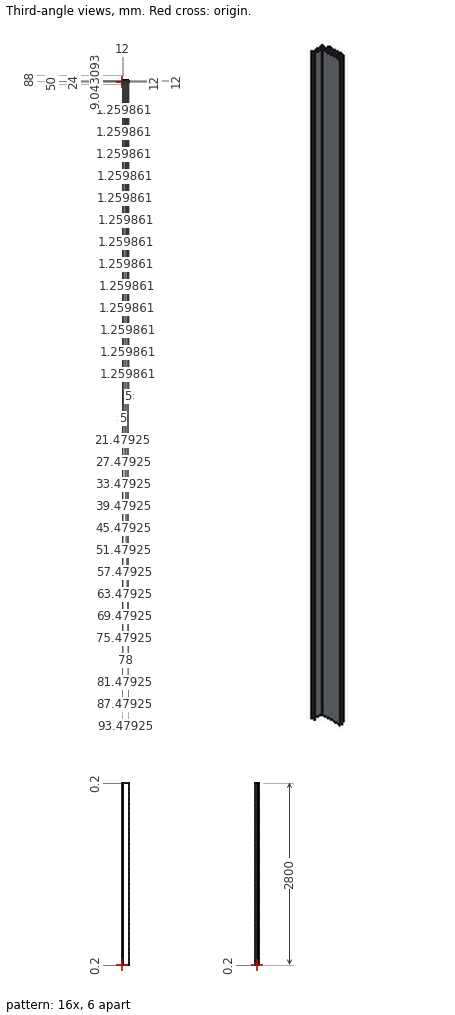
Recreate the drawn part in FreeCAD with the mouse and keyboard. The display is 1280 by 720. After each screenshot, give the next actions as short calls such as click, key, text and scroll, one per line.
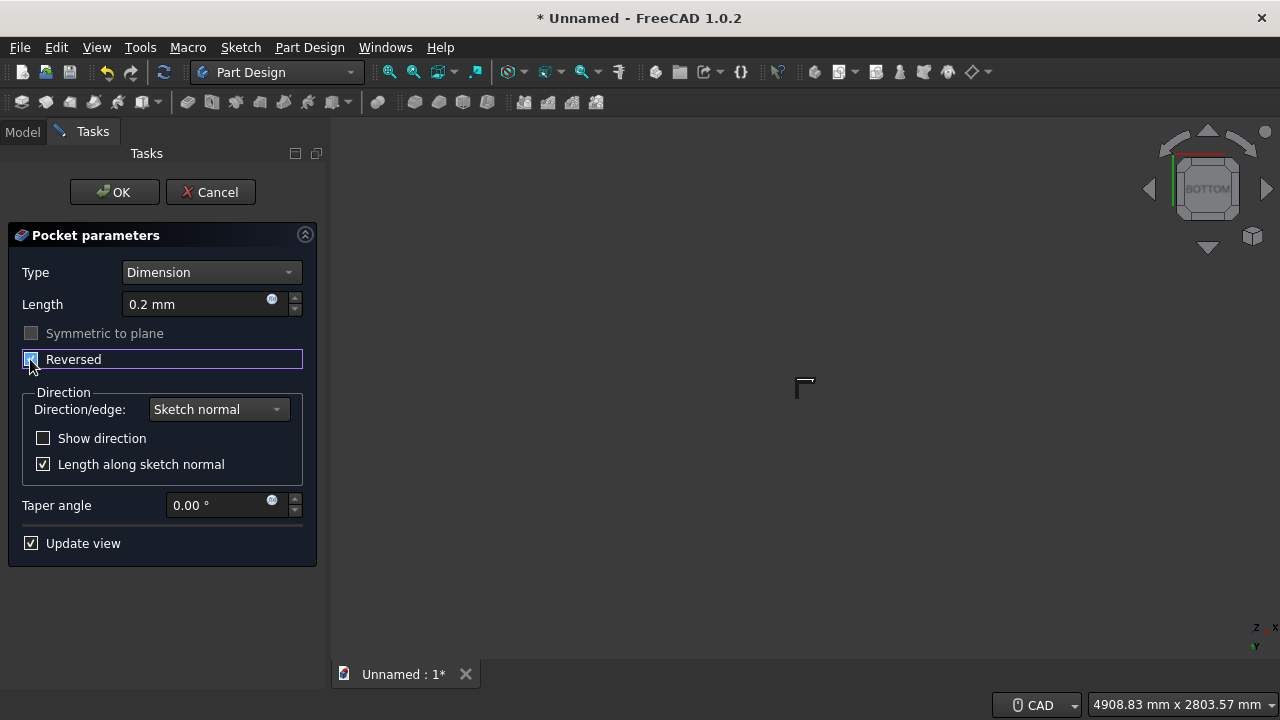
click(115, 192)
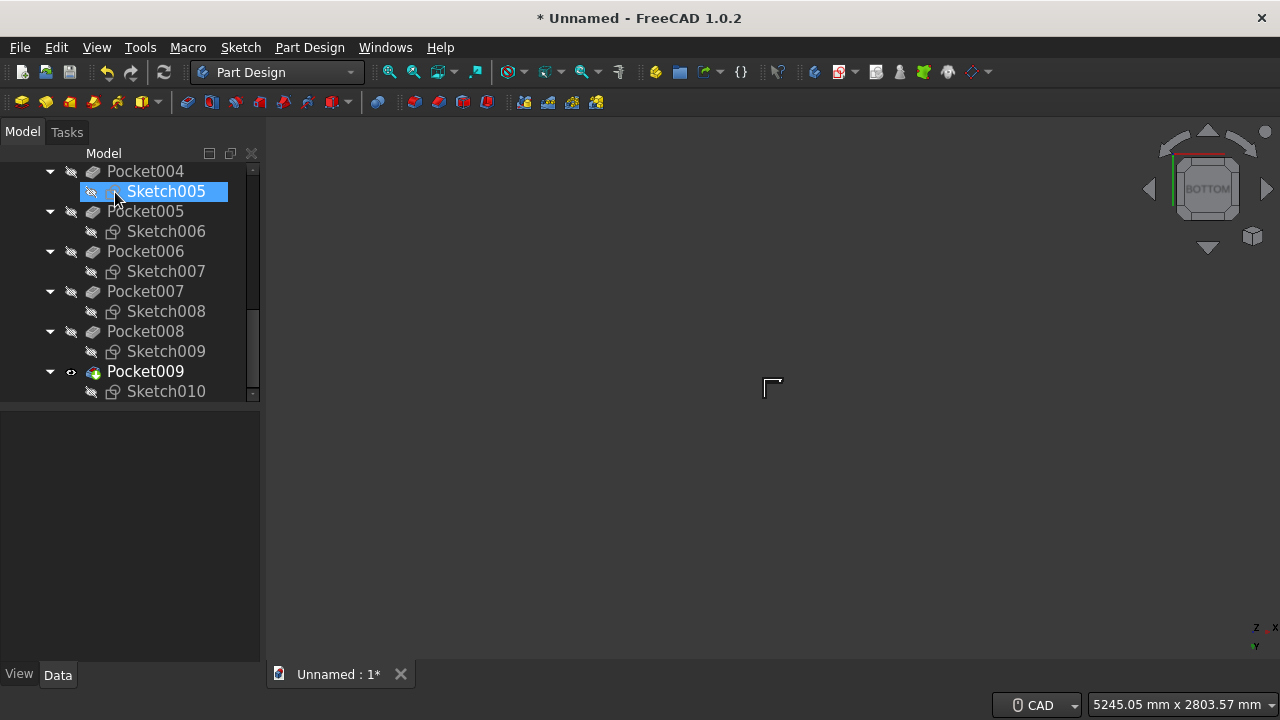
click(390, 72)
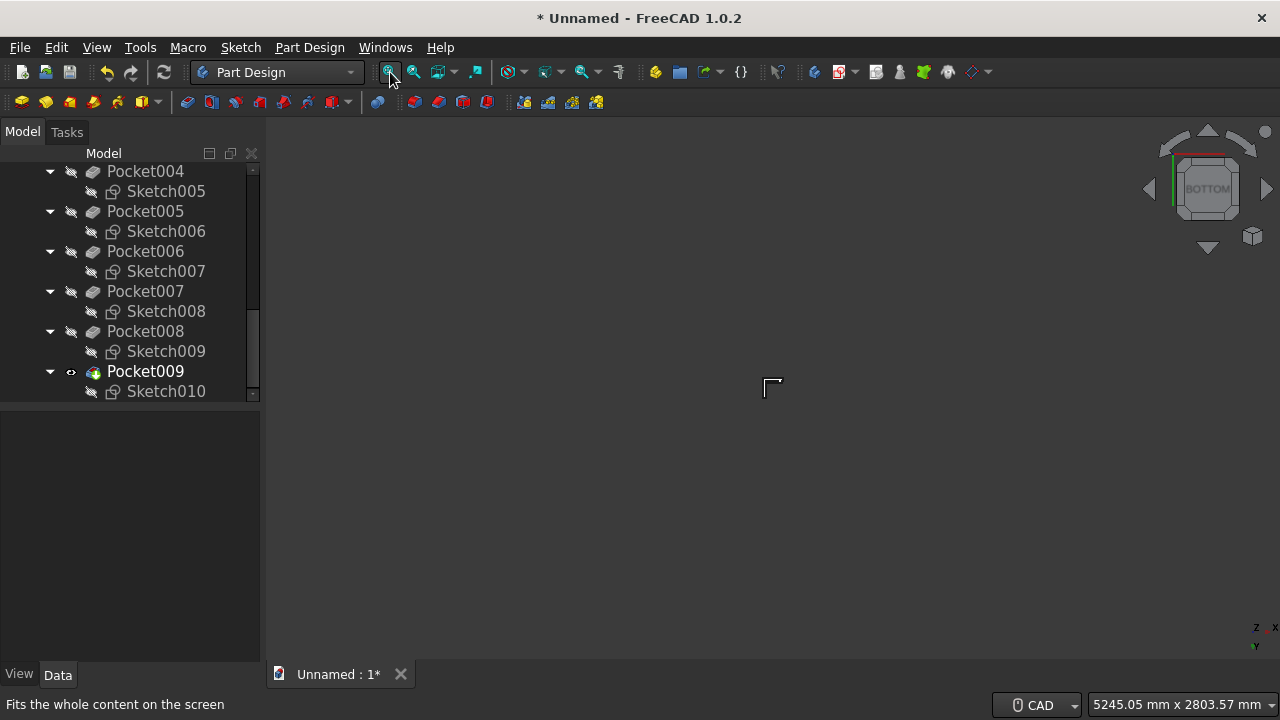
scroll(779, 379, up, 11)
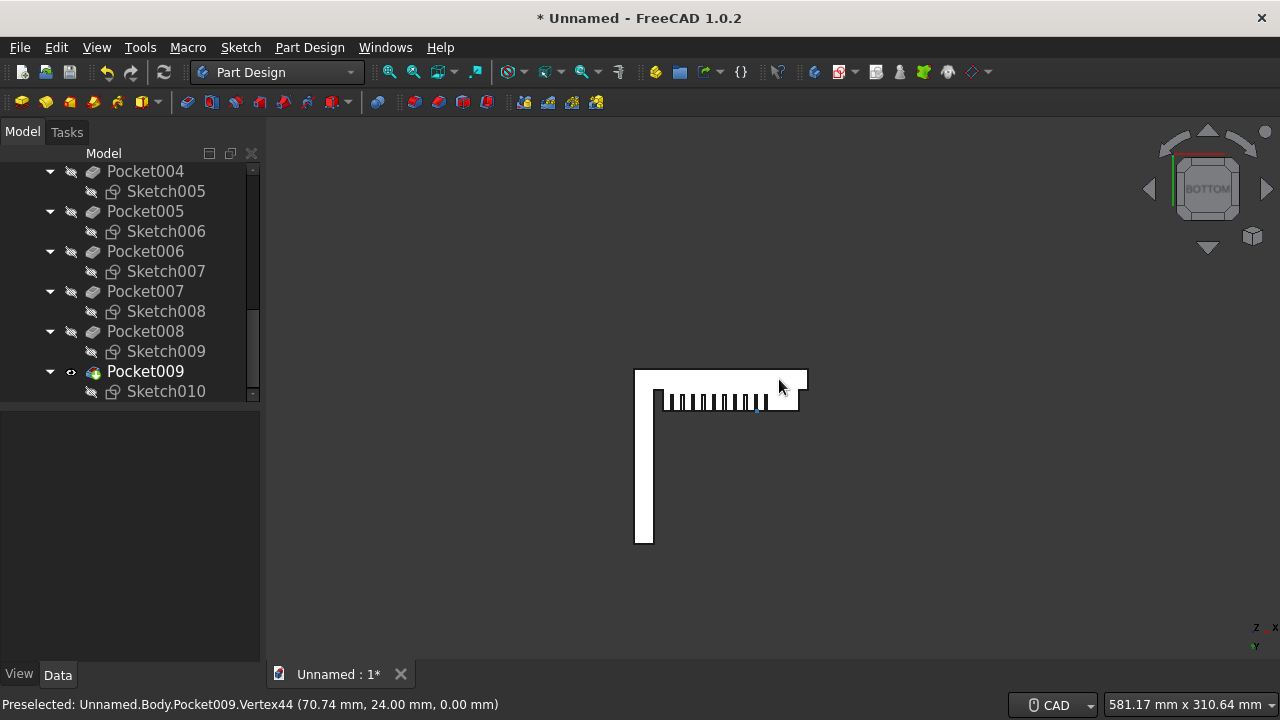
click(771, 381)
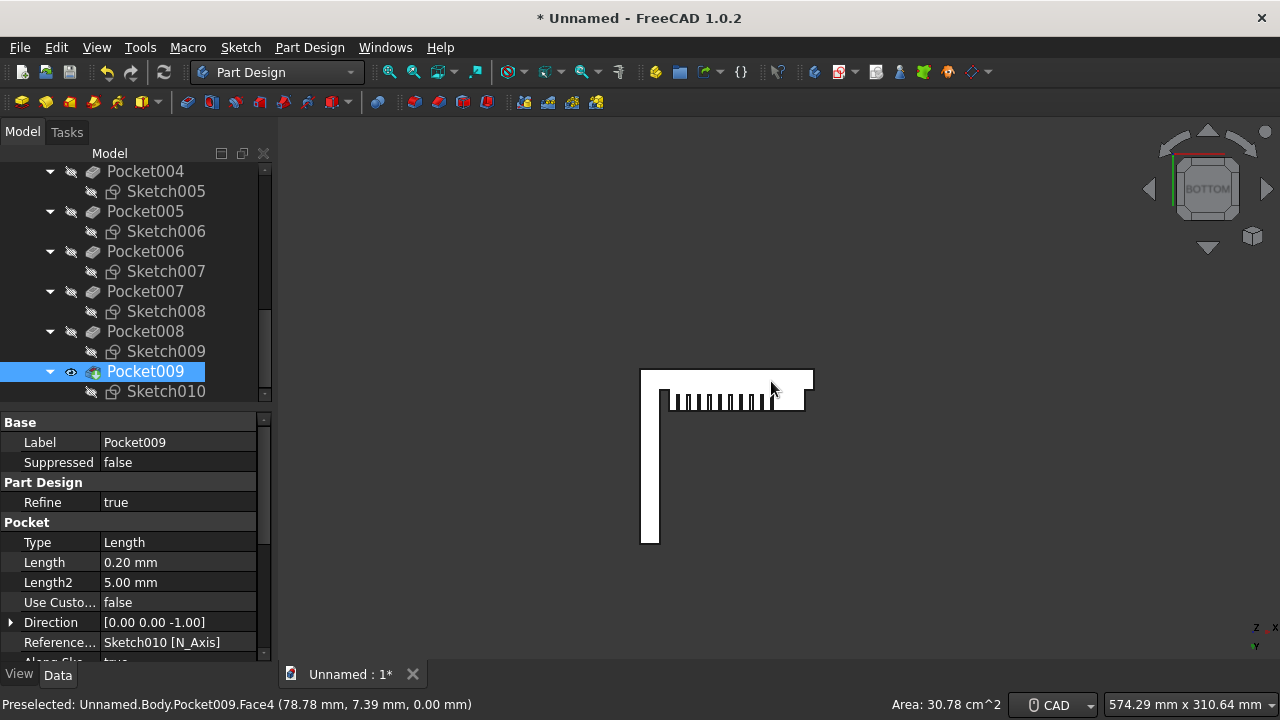
click(840, 72)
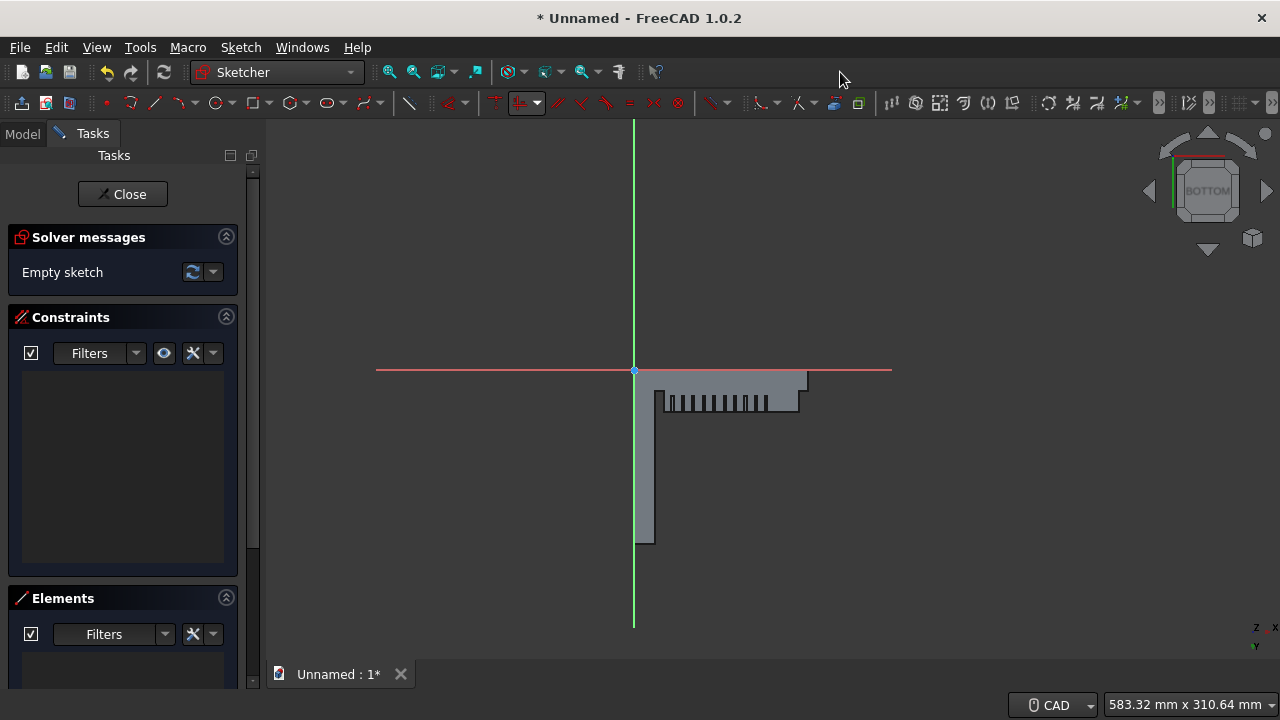
scroll(781, 405, up, 15)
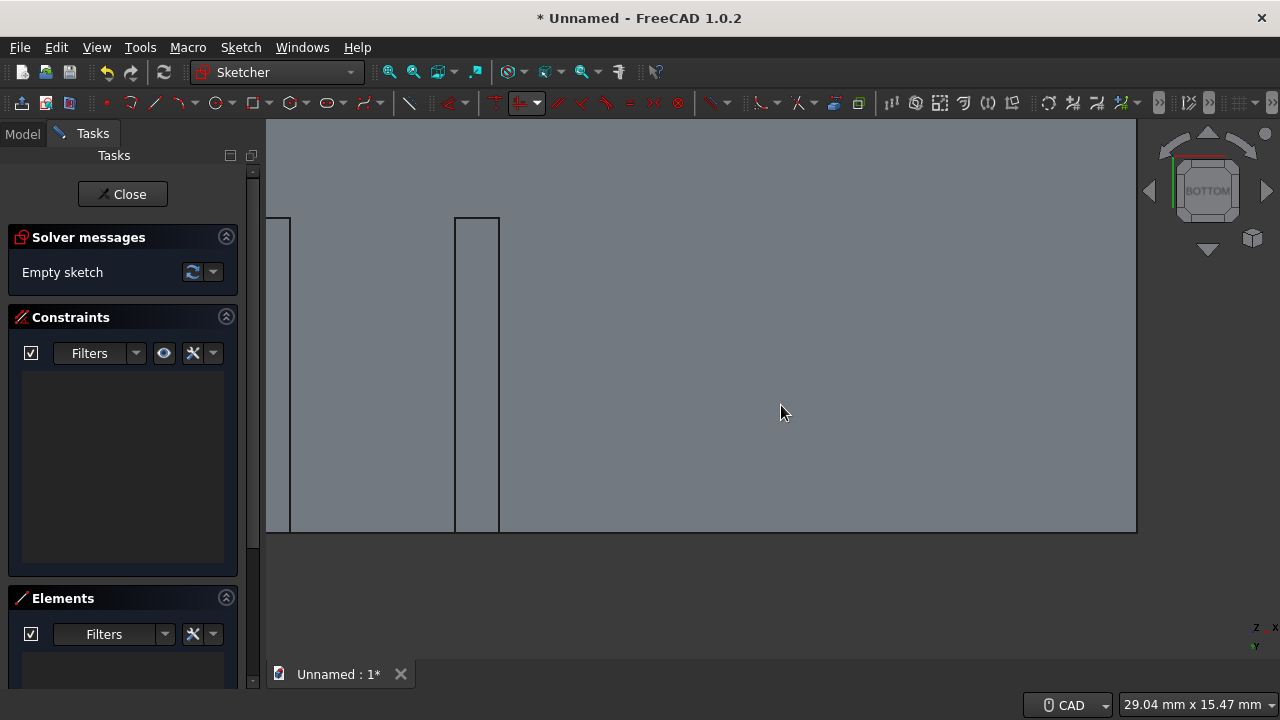
click(254, 104)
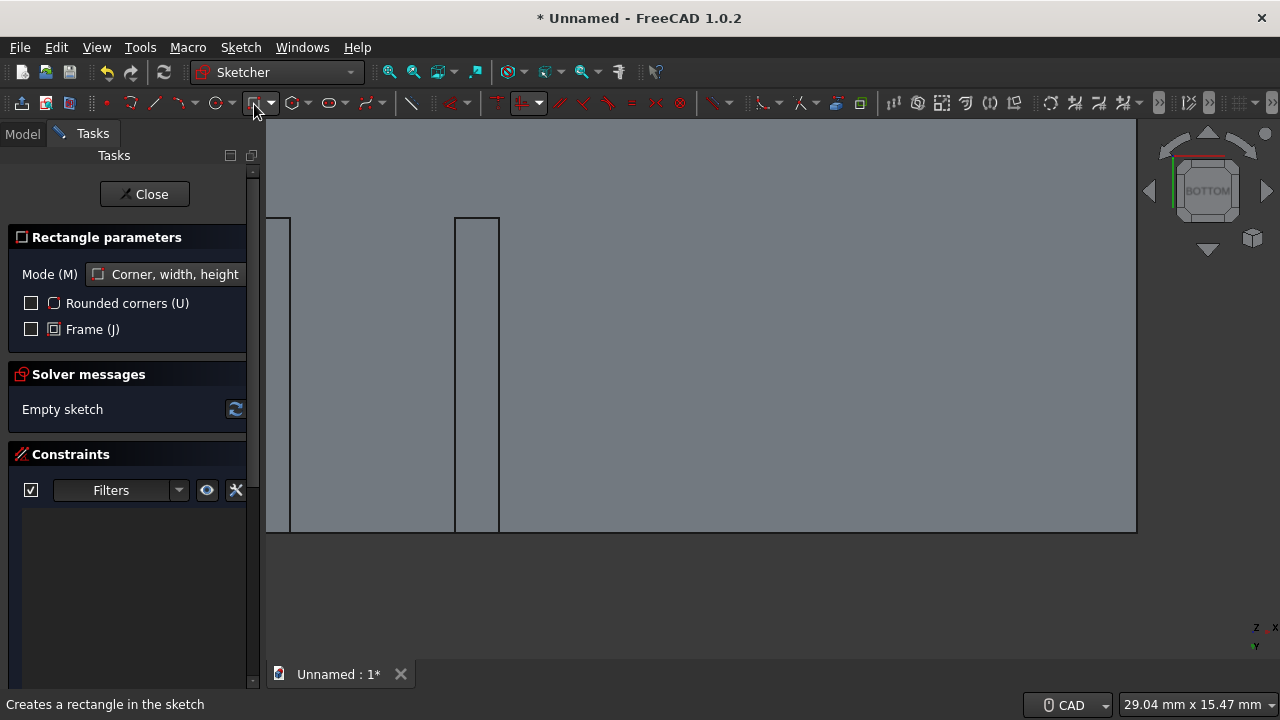
click(665, 218)
move(709, 533)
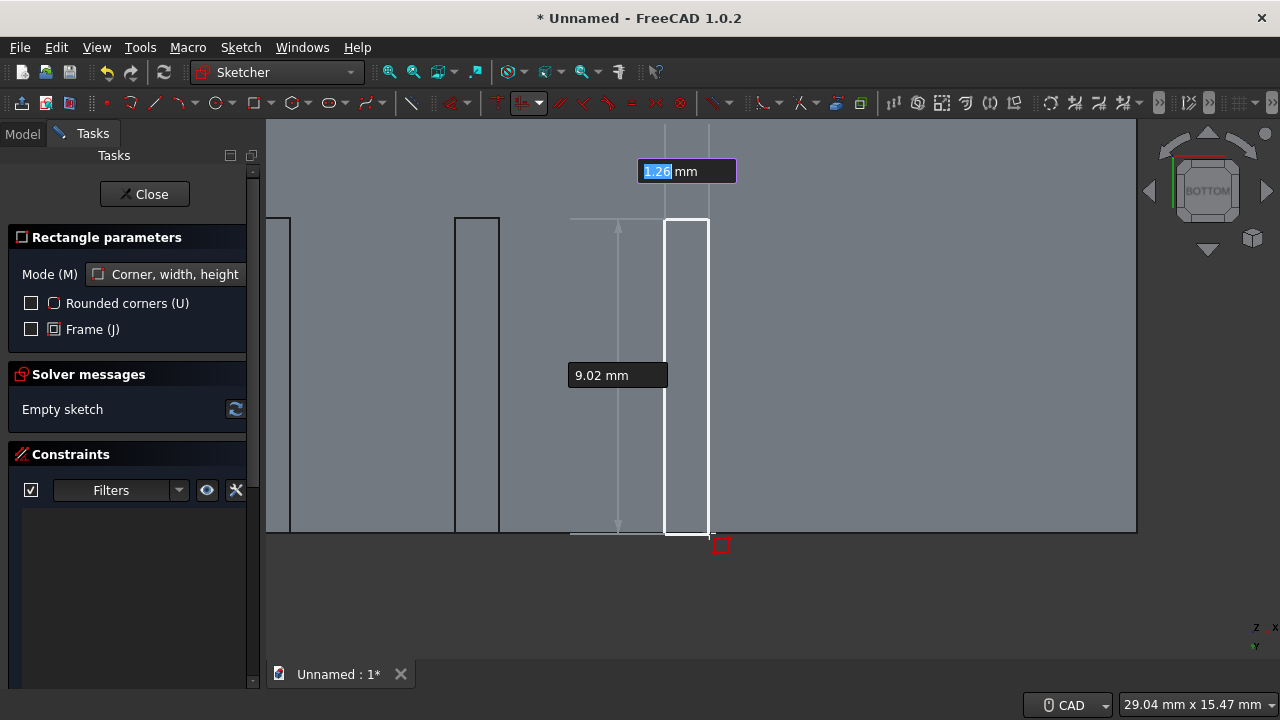
text(1.259861)
key(Tab)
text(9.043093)
key(Return)
key(Escape)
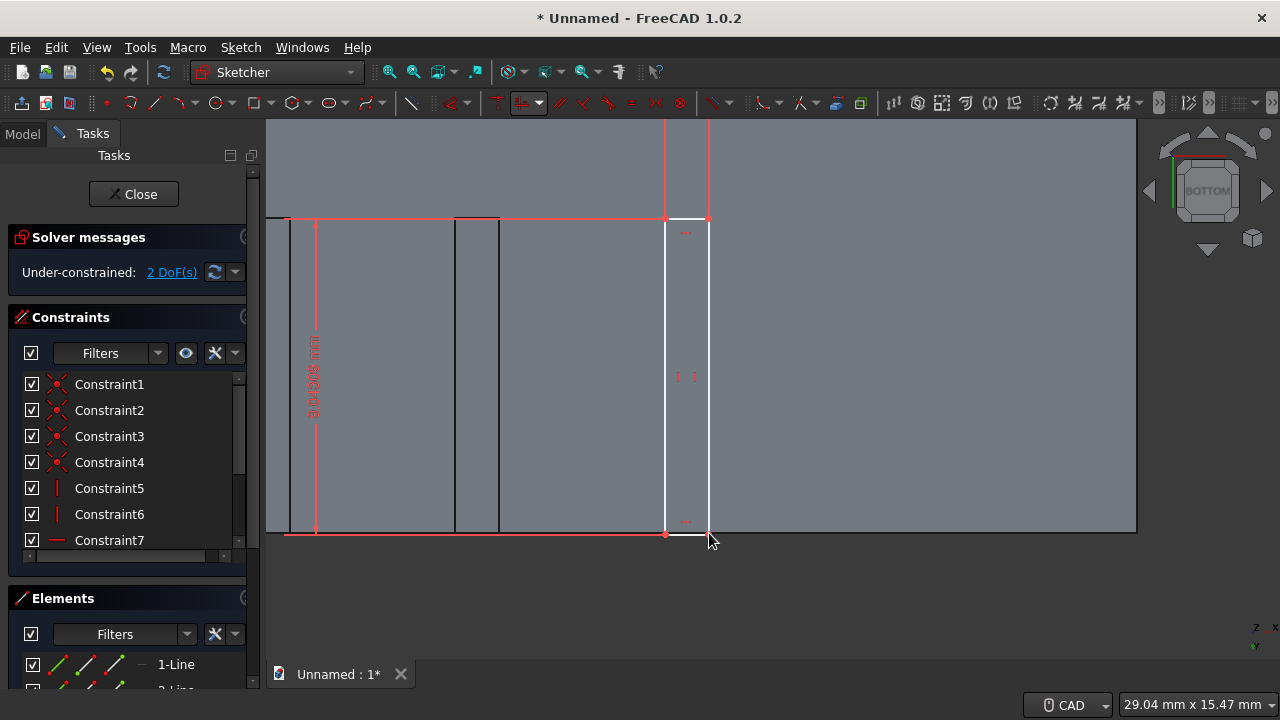
click(450, 104)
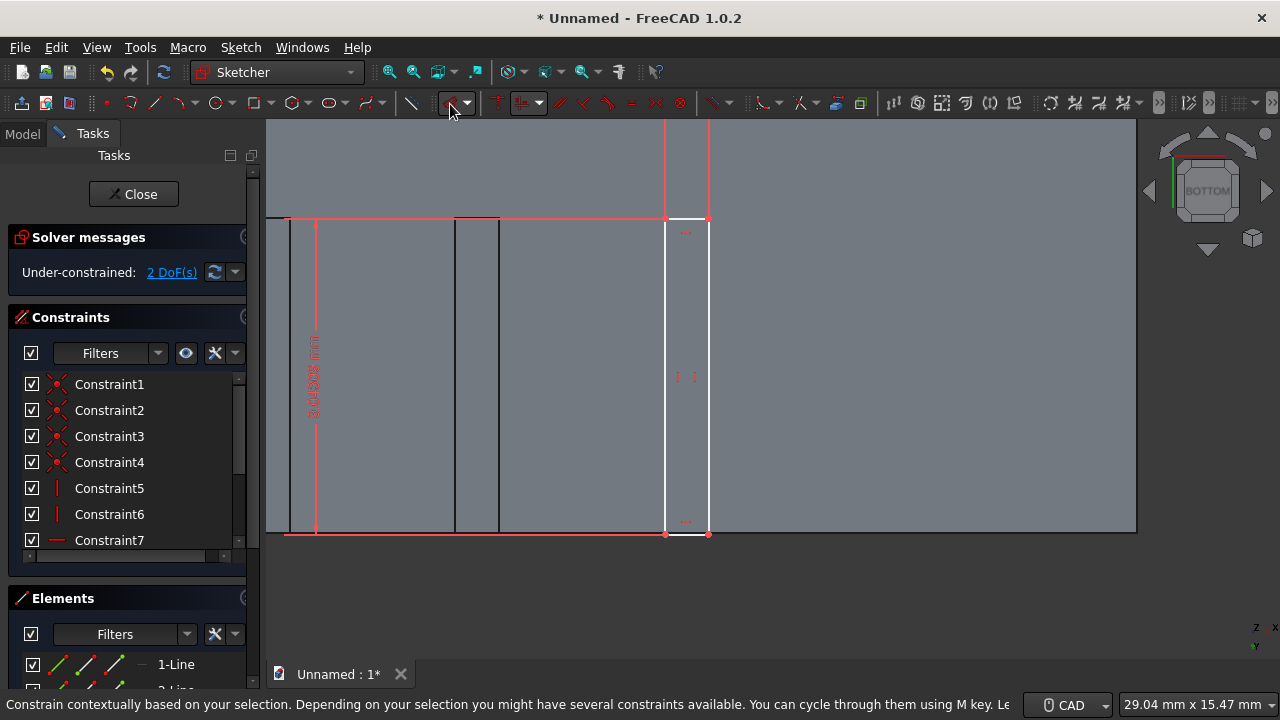
click(665, 535)
click(699, 205)